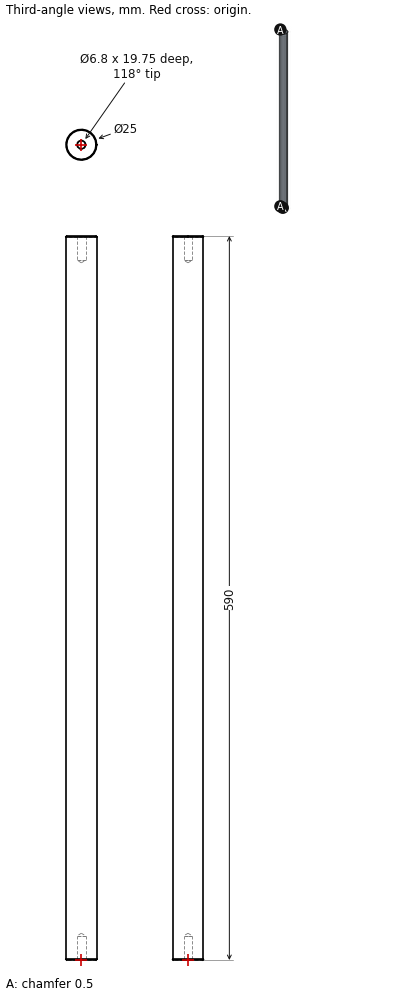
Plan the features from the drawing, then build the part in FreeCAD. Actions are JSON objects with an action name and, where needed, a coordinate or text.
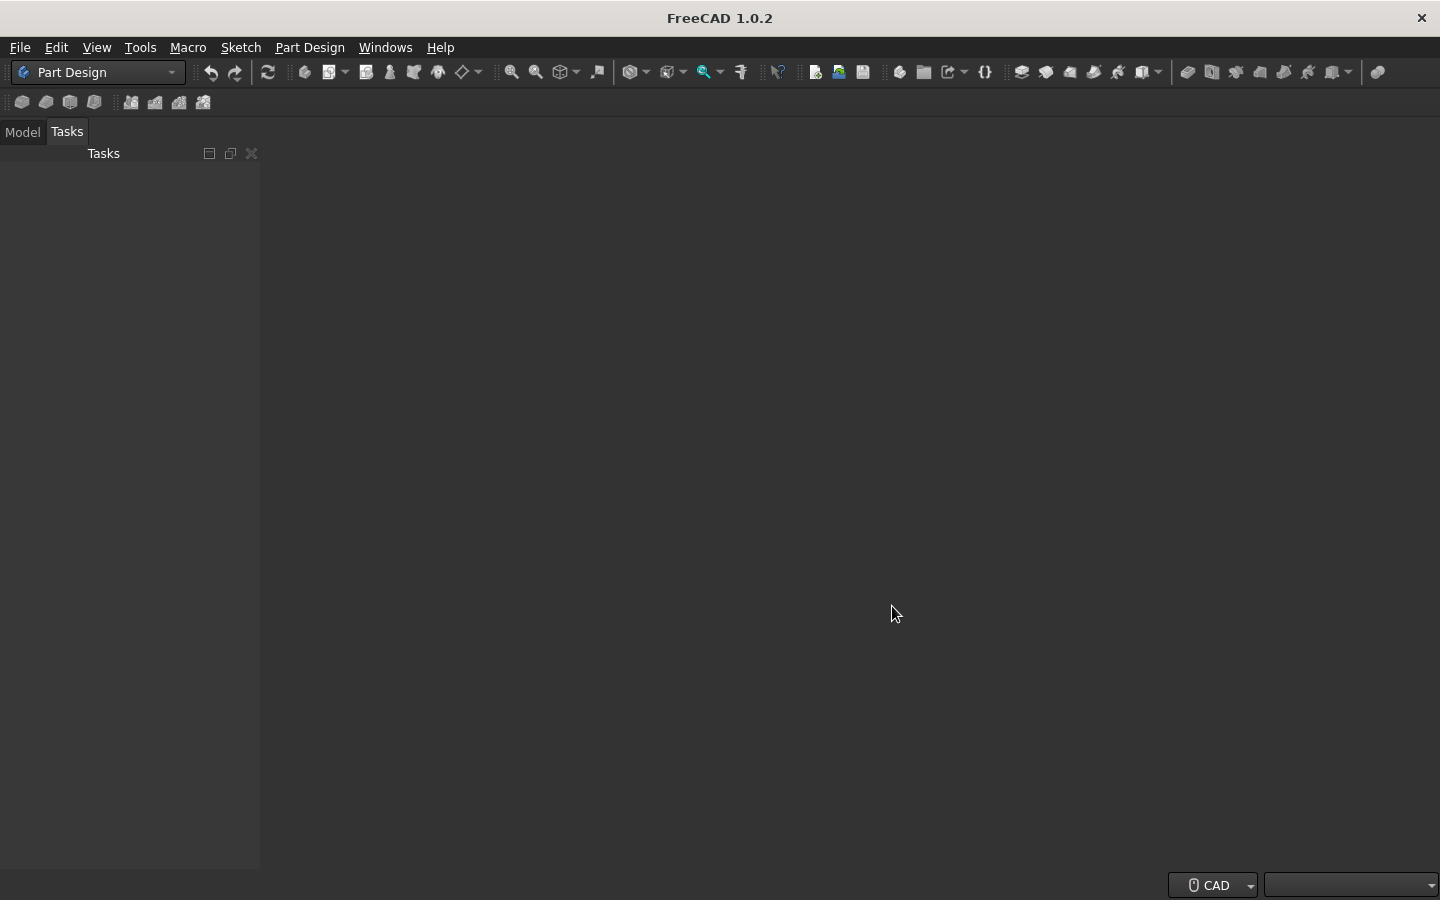
{"action": "key", "text": "ctrl+n"}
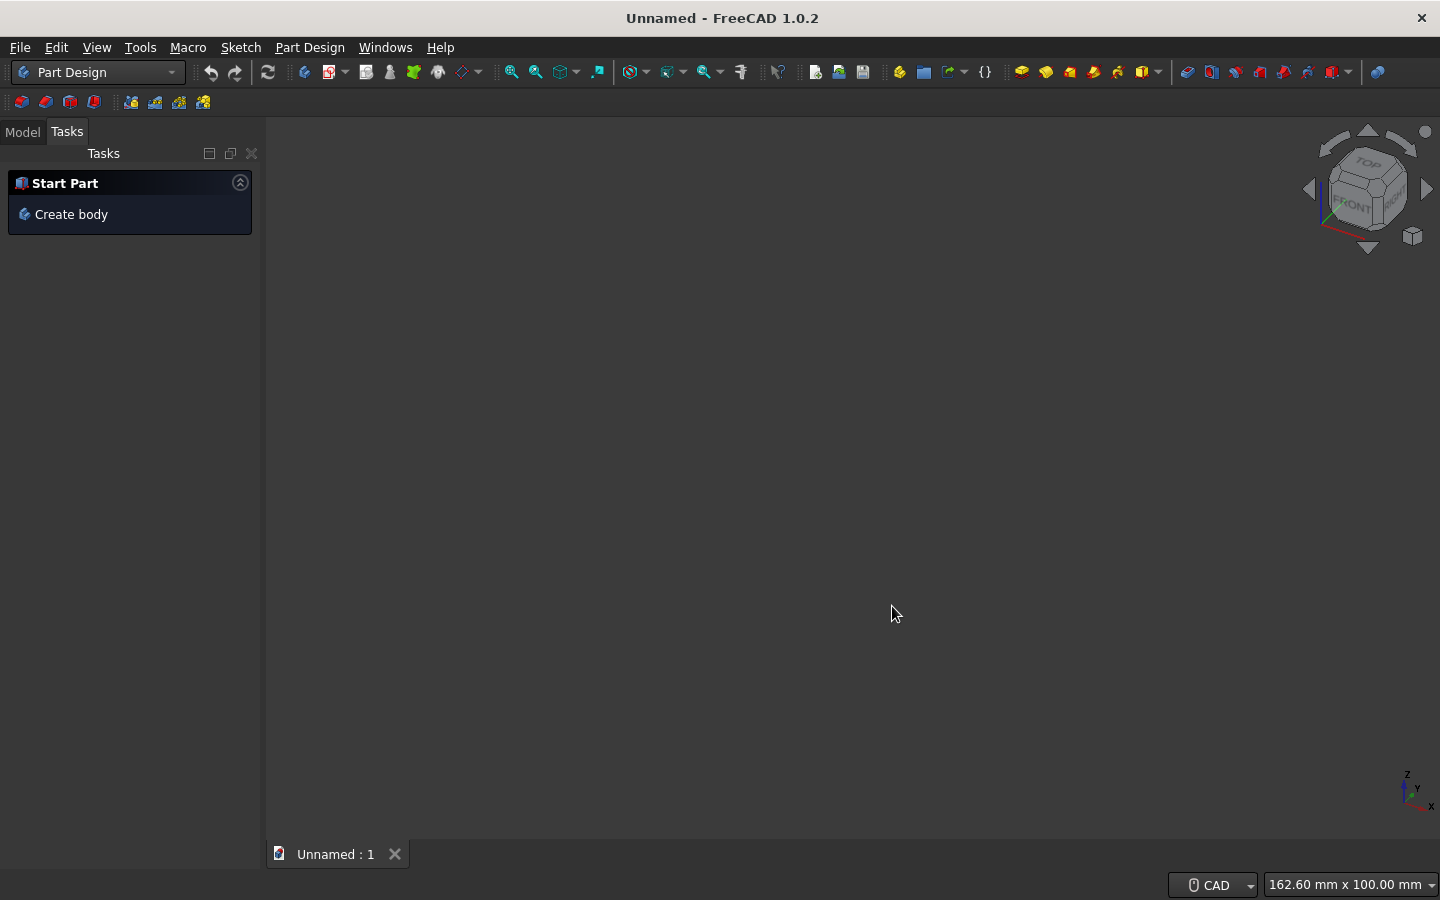
{"action": "left_click", "coordinate": [330, 72]}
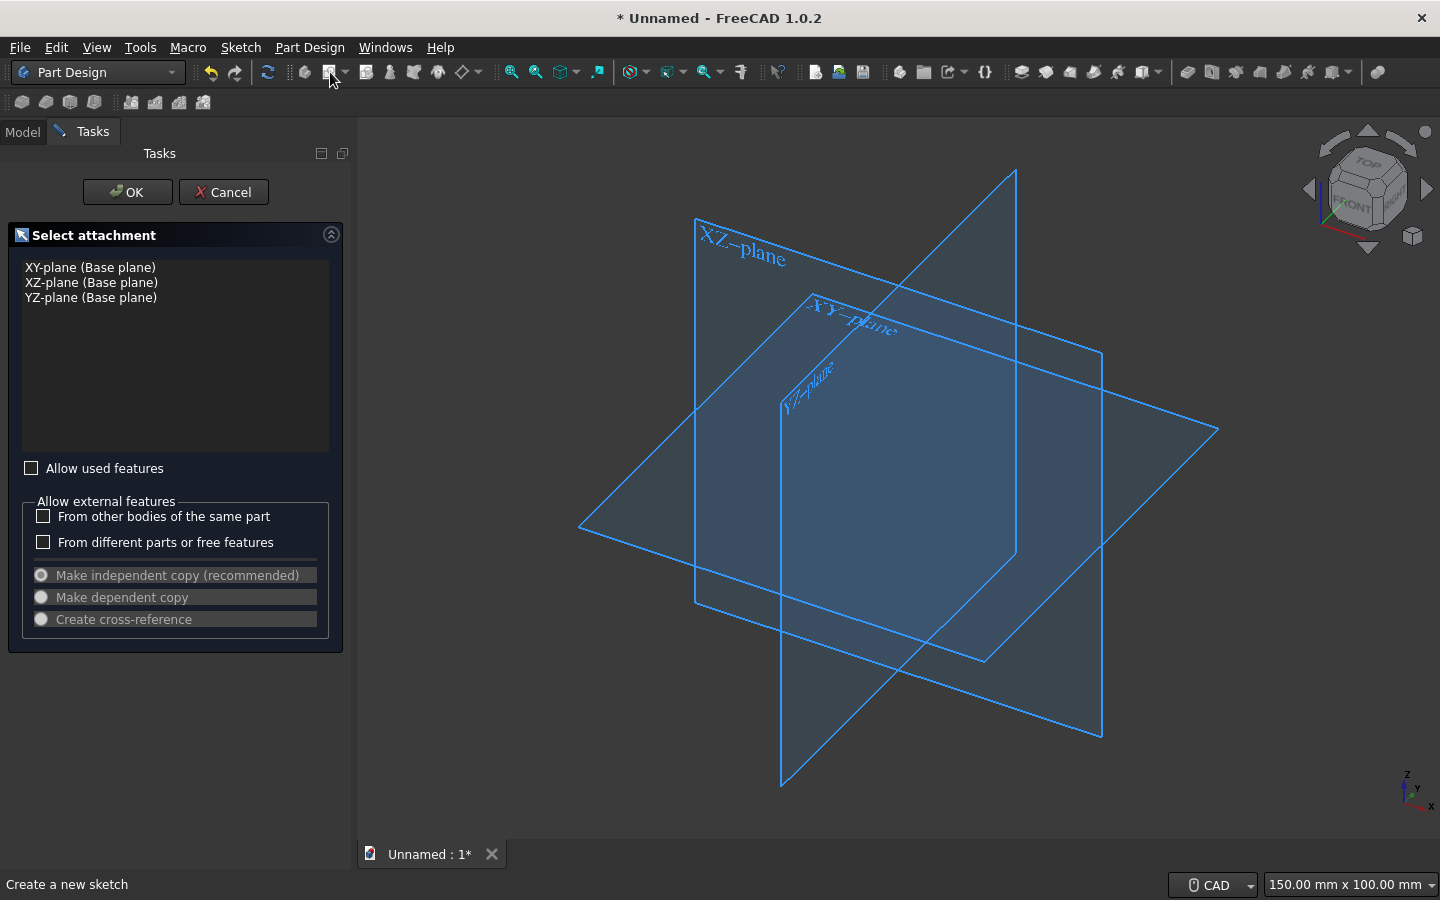
{"action": "left_click", "coordinate": [82, 268]}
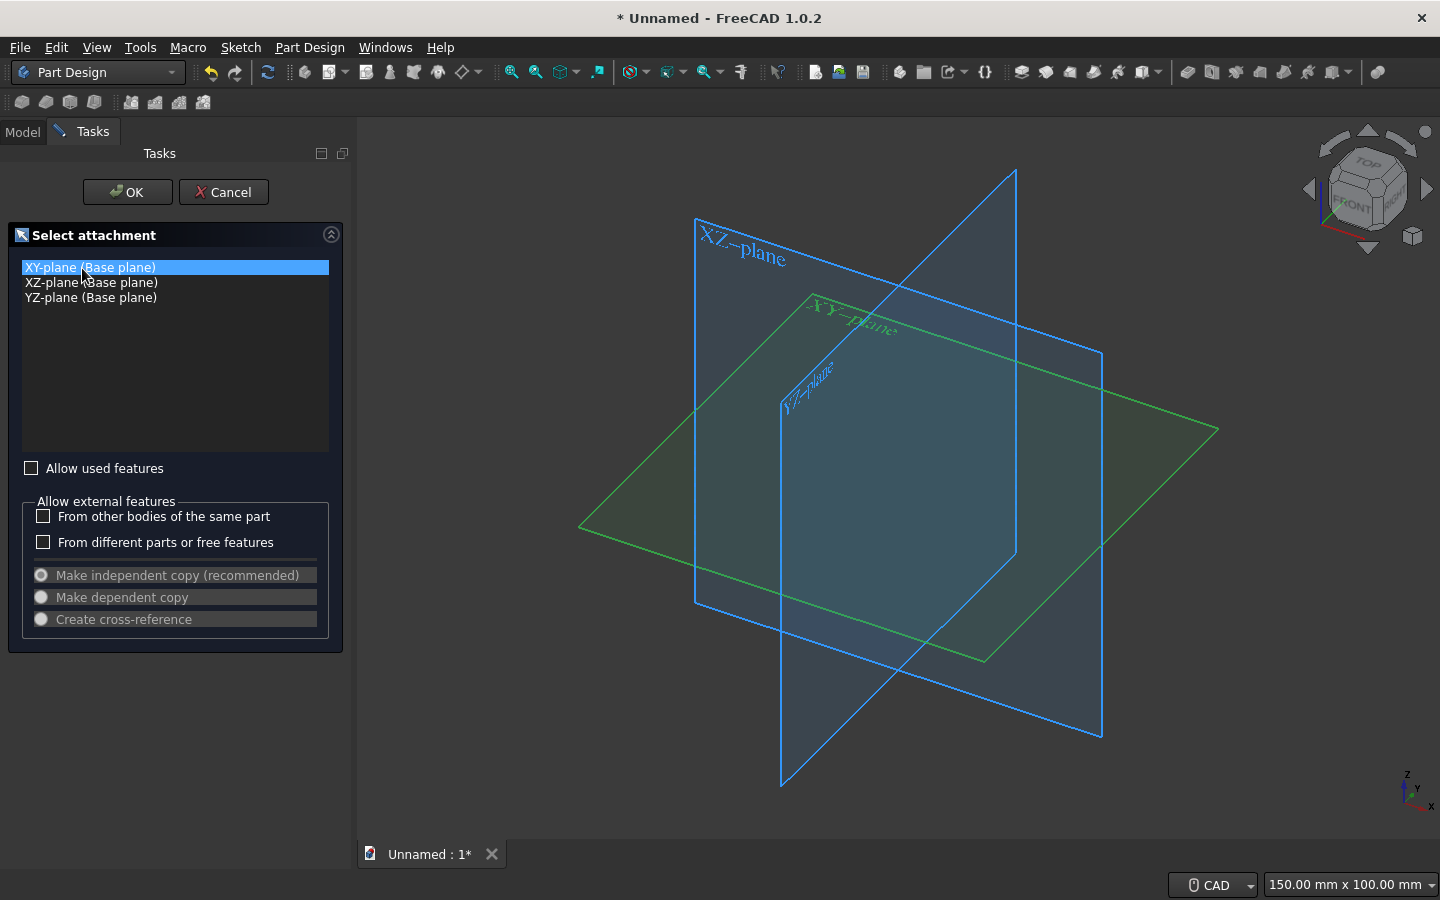
{"action": "left_click", "coordinate": [128, 192]}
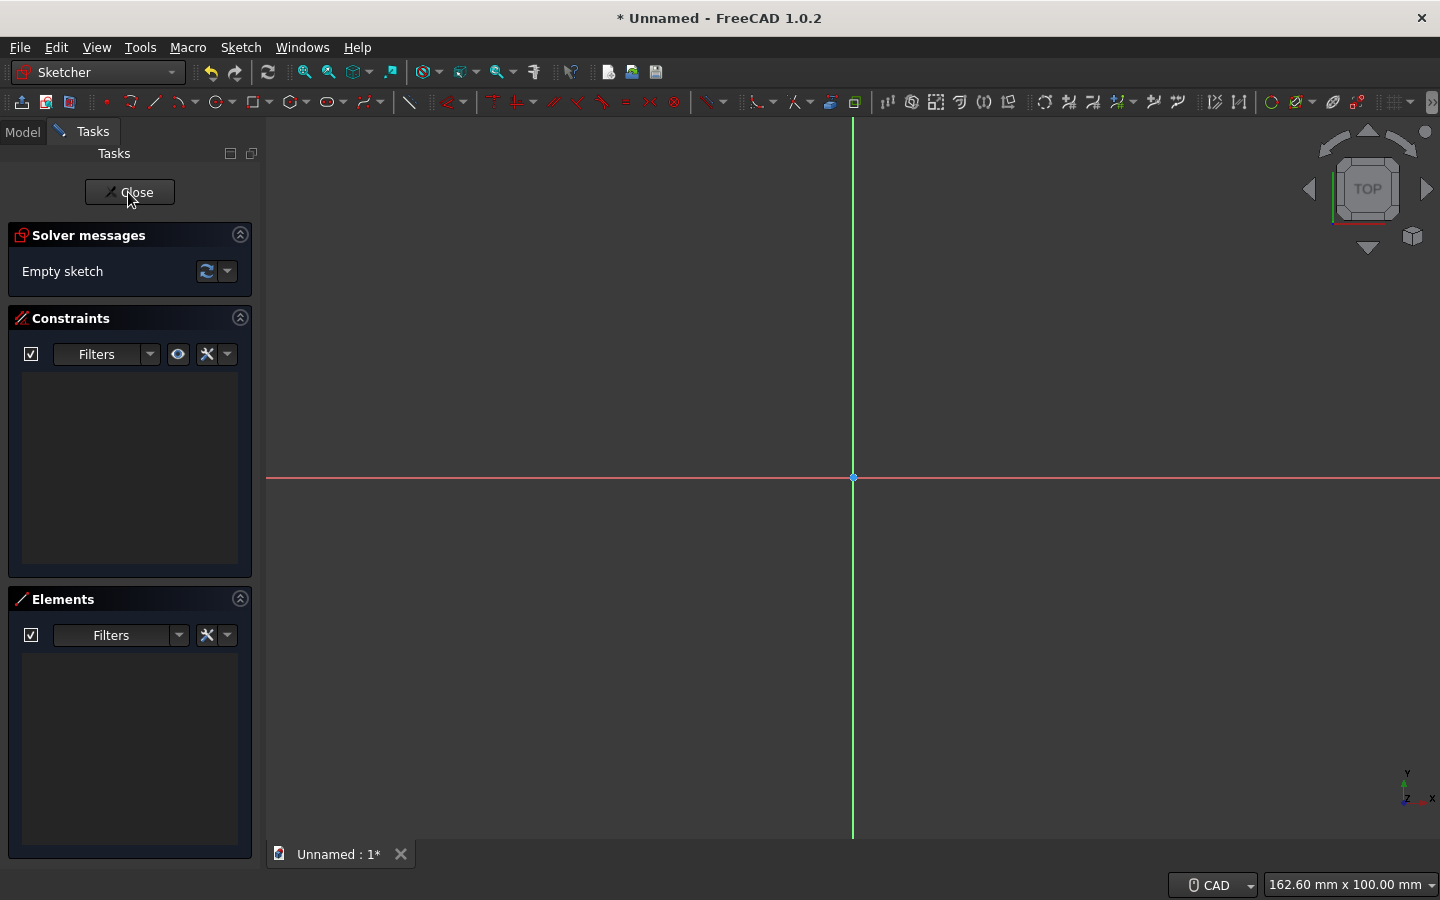
{"action": "scroll", "coordinate": [893, 478], "scroll_direction": "up", "scroll_amount": 5}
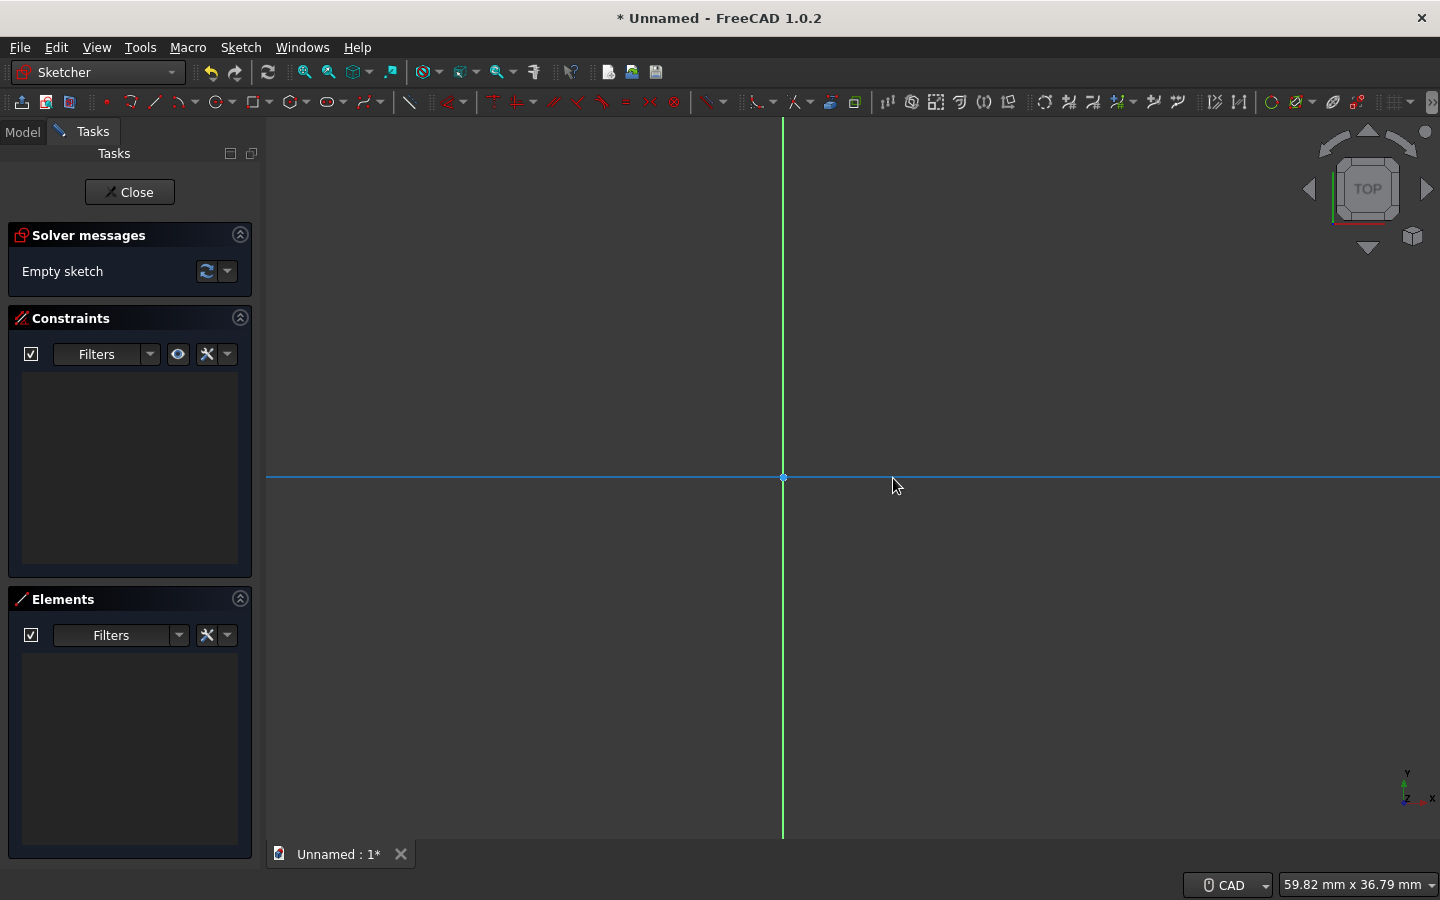
{"action": "key", "text": "g c"}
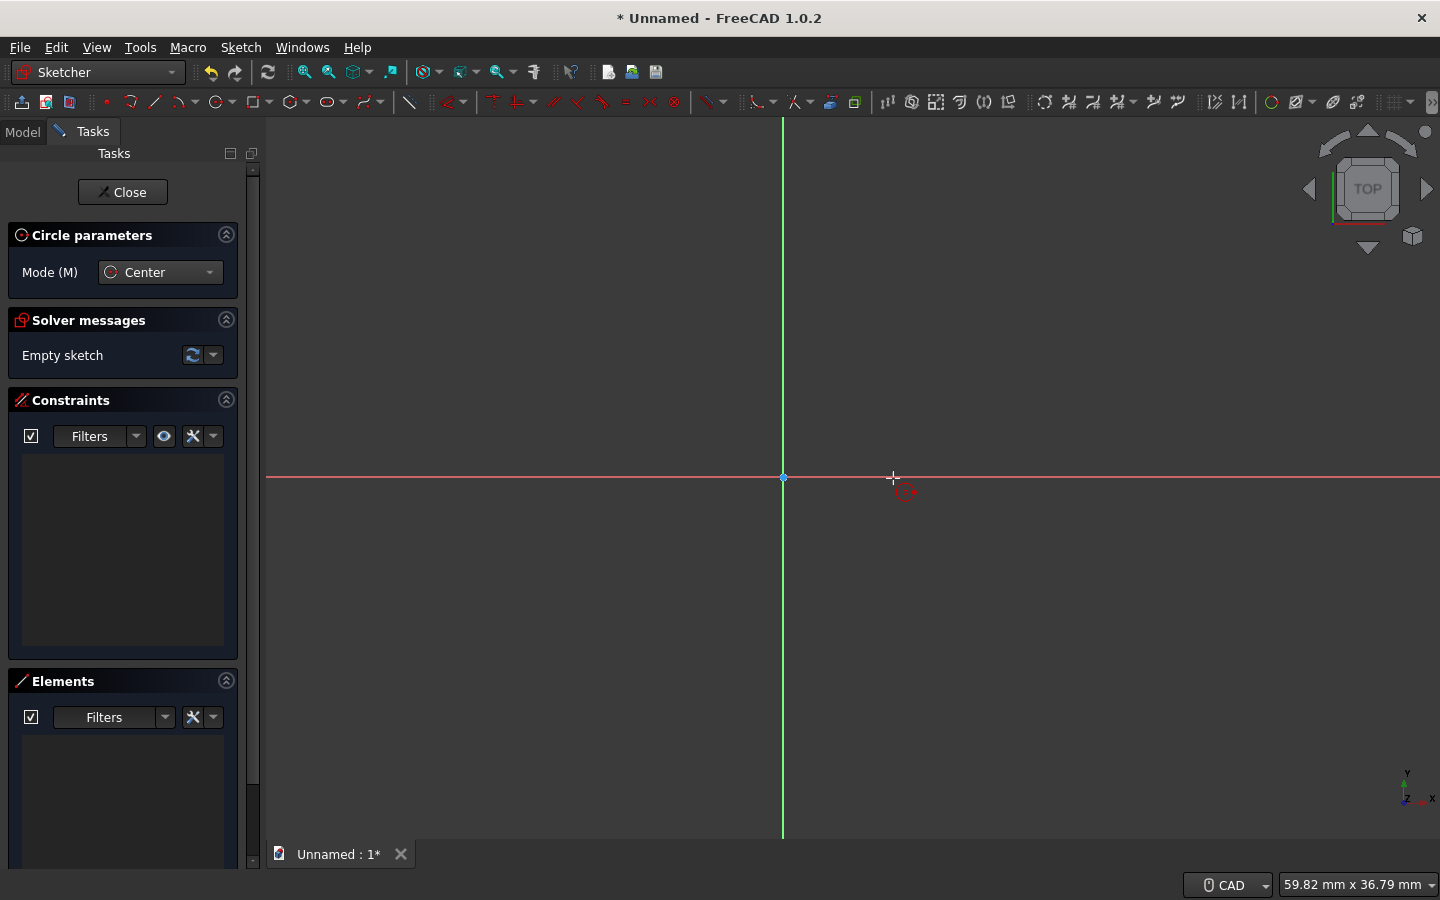
{"action": "left_click", "coordinate": [783, 477]}
{"action": "mouse_move", "coordinate": [957, 304]}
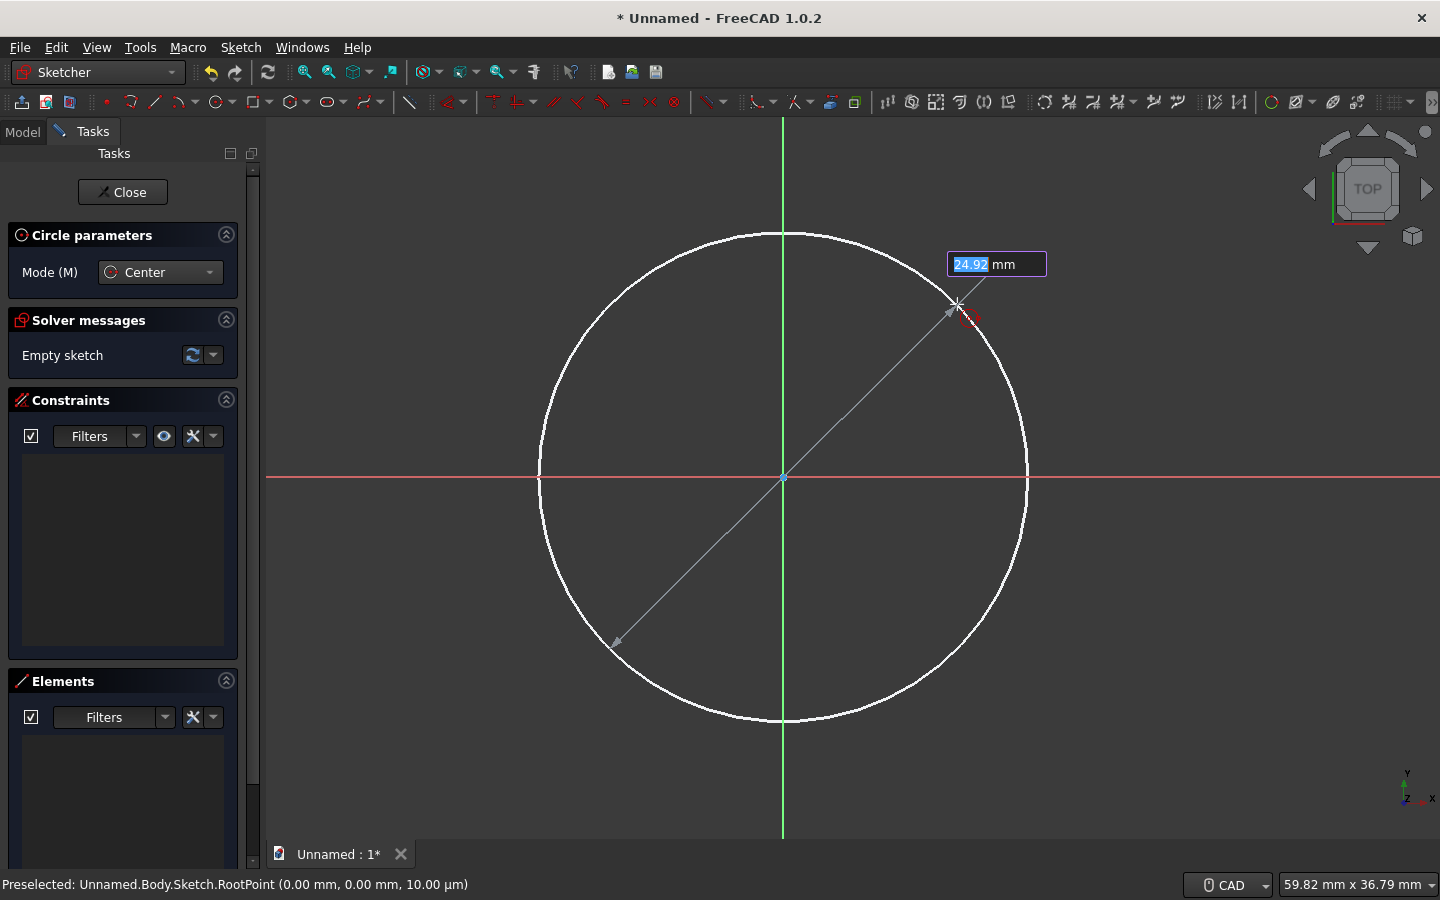
{"action": "type", "text": "25"}
{"action": "key", "text": "Return"}
{"action": "key", "text": "Escape"}